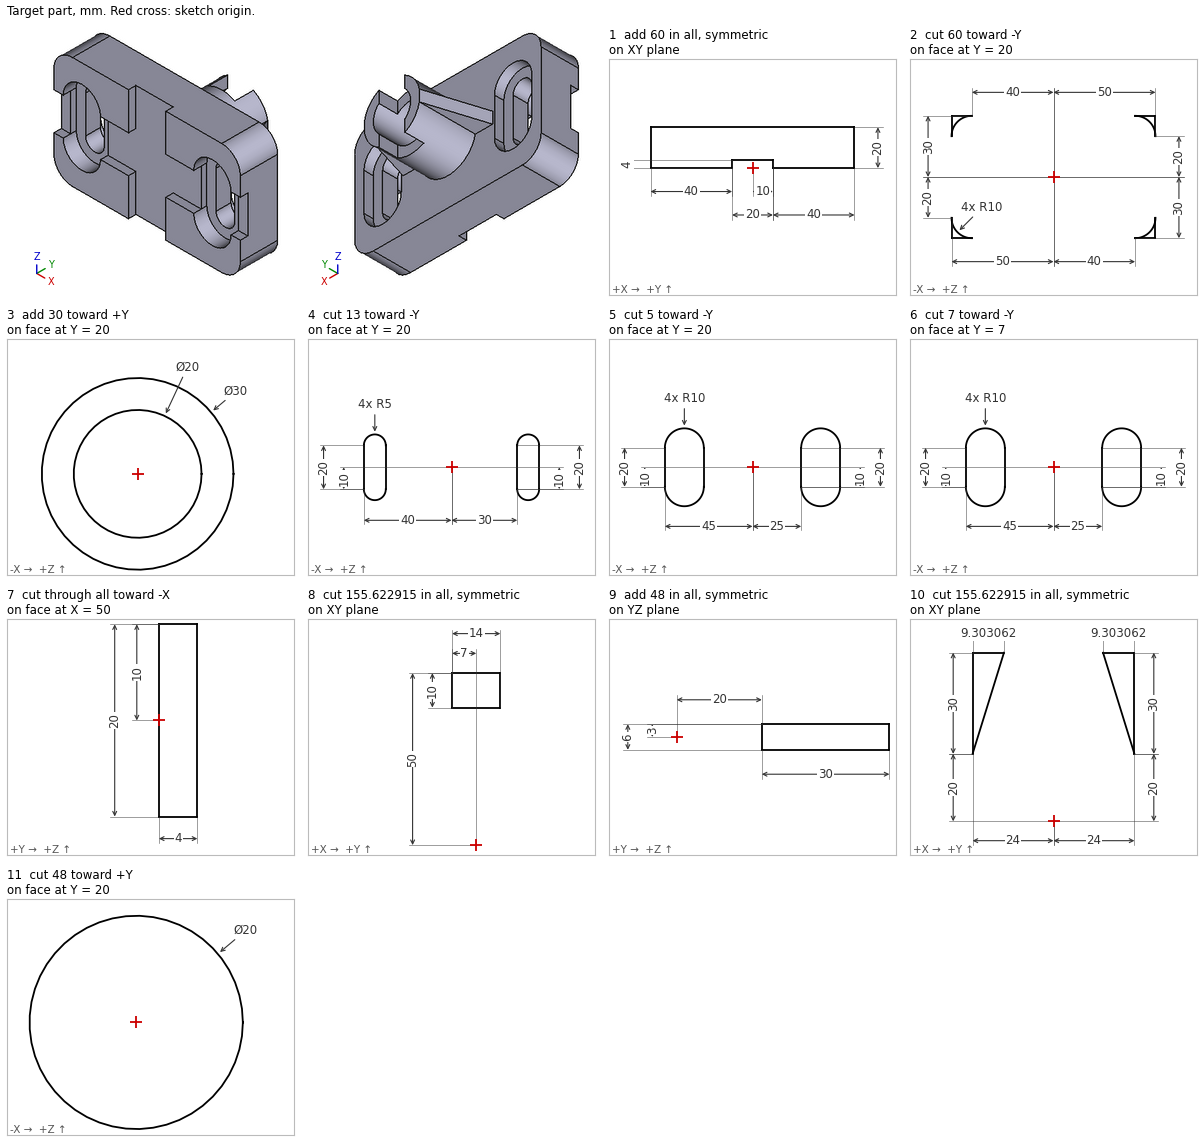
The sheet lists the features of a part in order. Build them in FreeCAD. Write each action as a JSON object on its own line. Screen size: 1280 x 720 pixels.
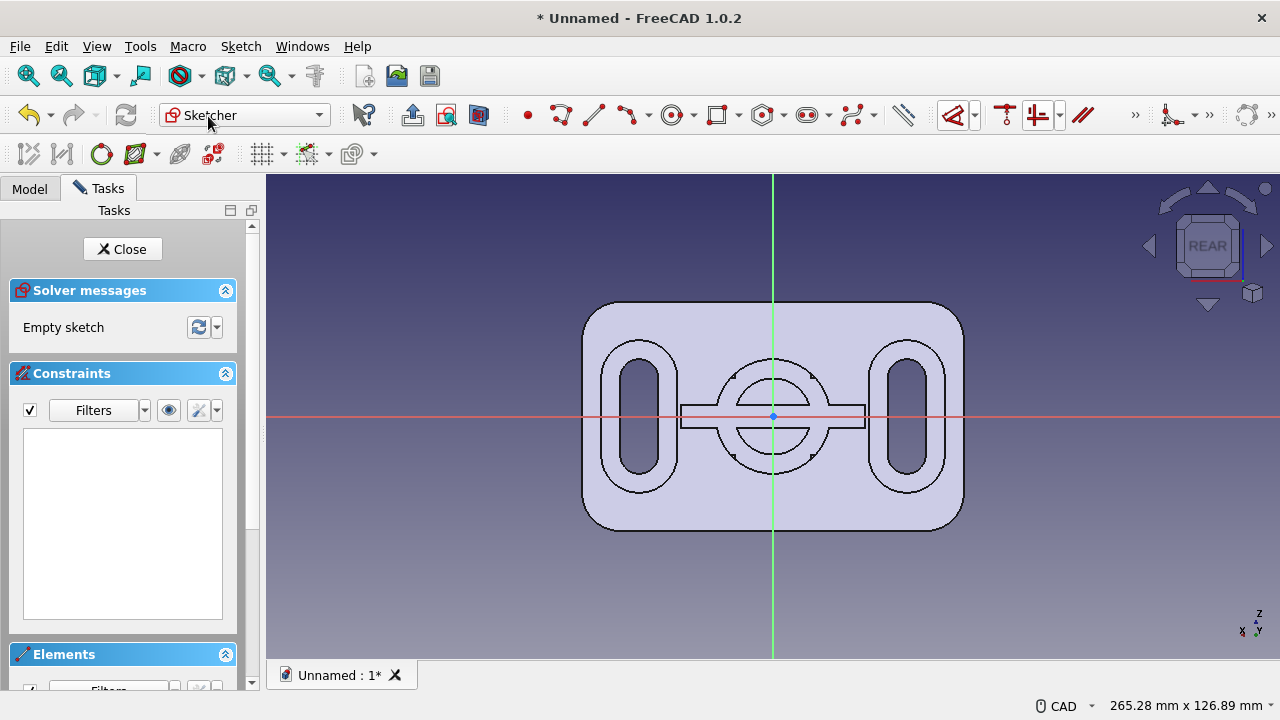
{"action": "scroll", "coordinate": [795, 416], "scroll_direction": "up", "scroll_amount": 7}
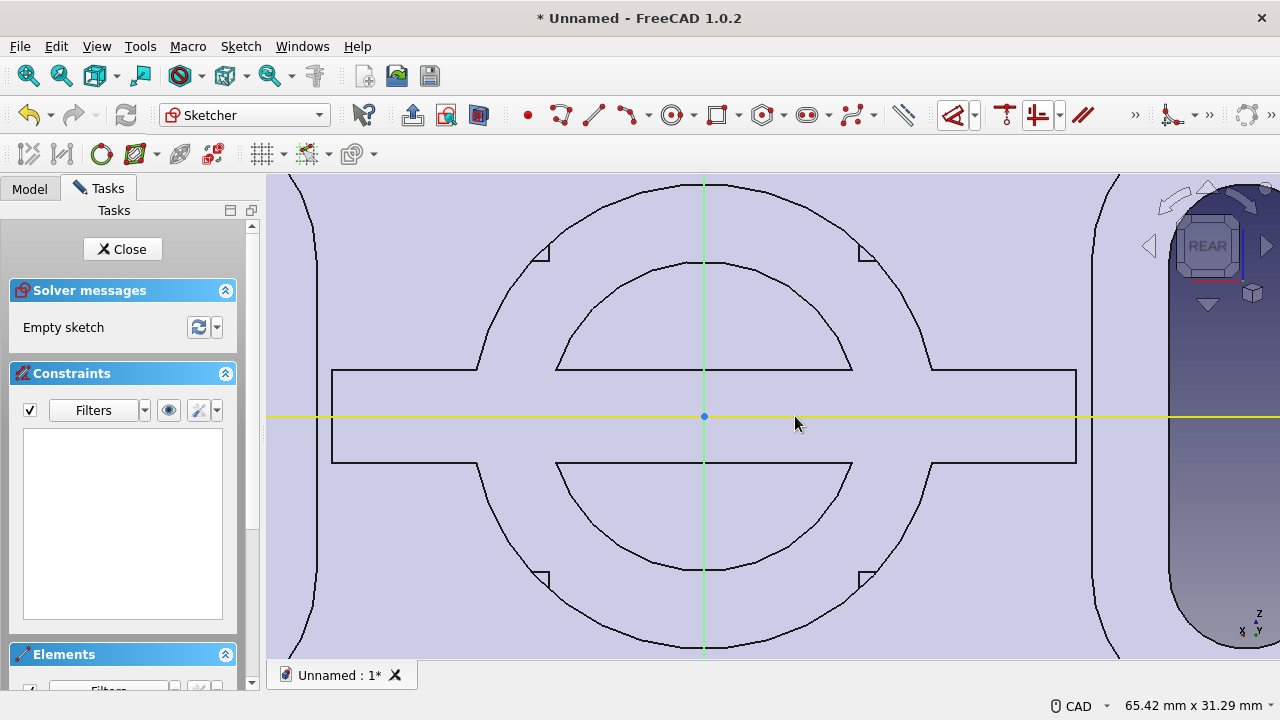
{"action": "key", "text": "g c"}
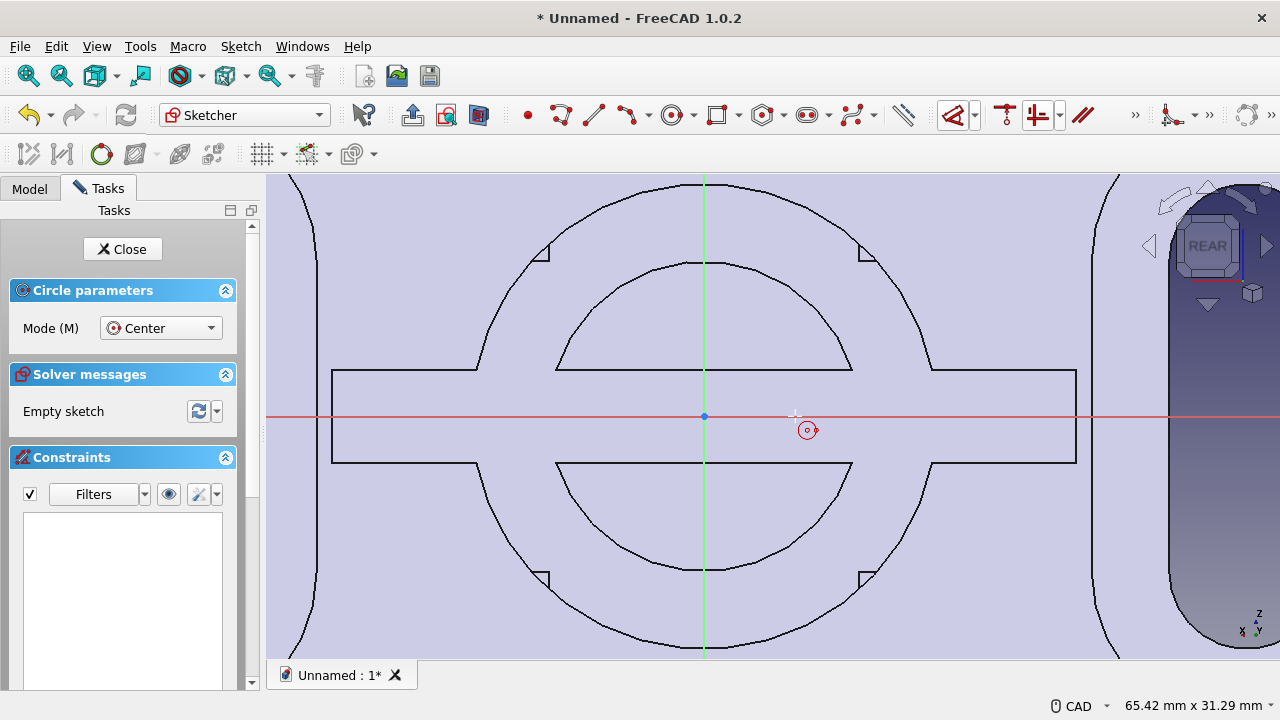
{"action": "left_click", "coordinate": [704, 416]}
{"action": "left_click", "coordinate": [814, 307]}
{"action": "key", "text": "Escape"}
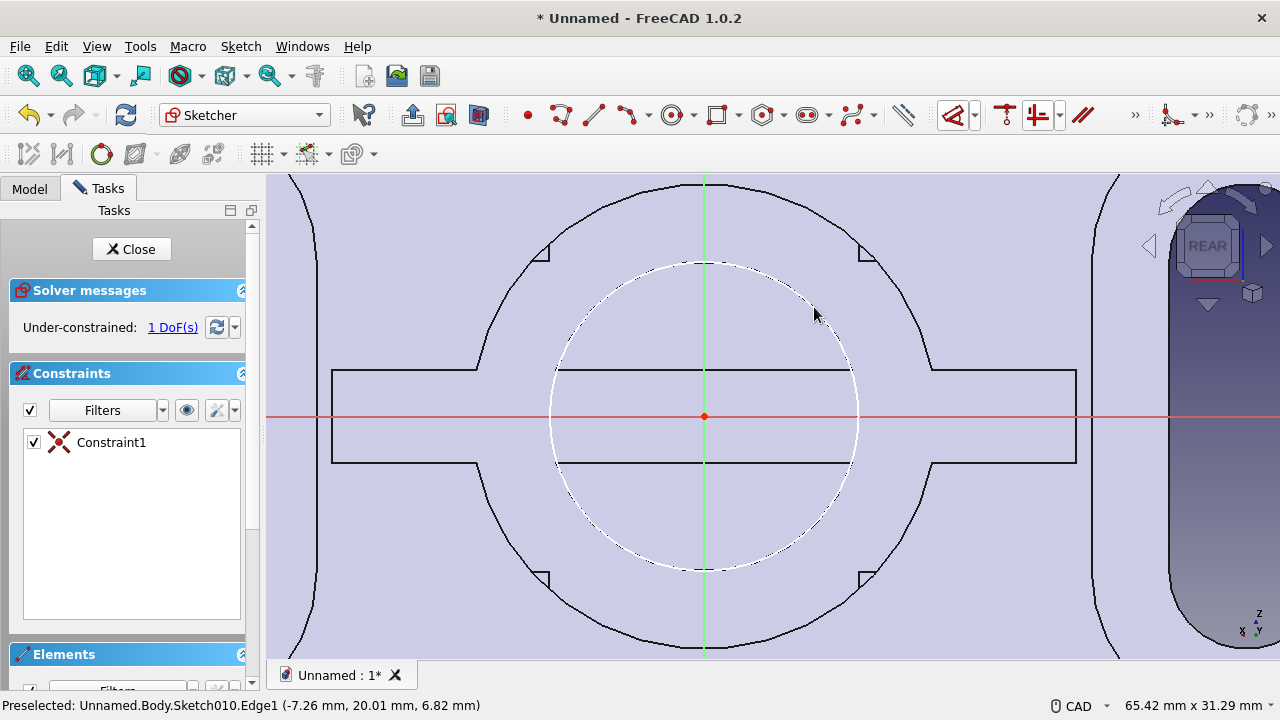
{"action": "left_click", "coordinate": [813, 307]}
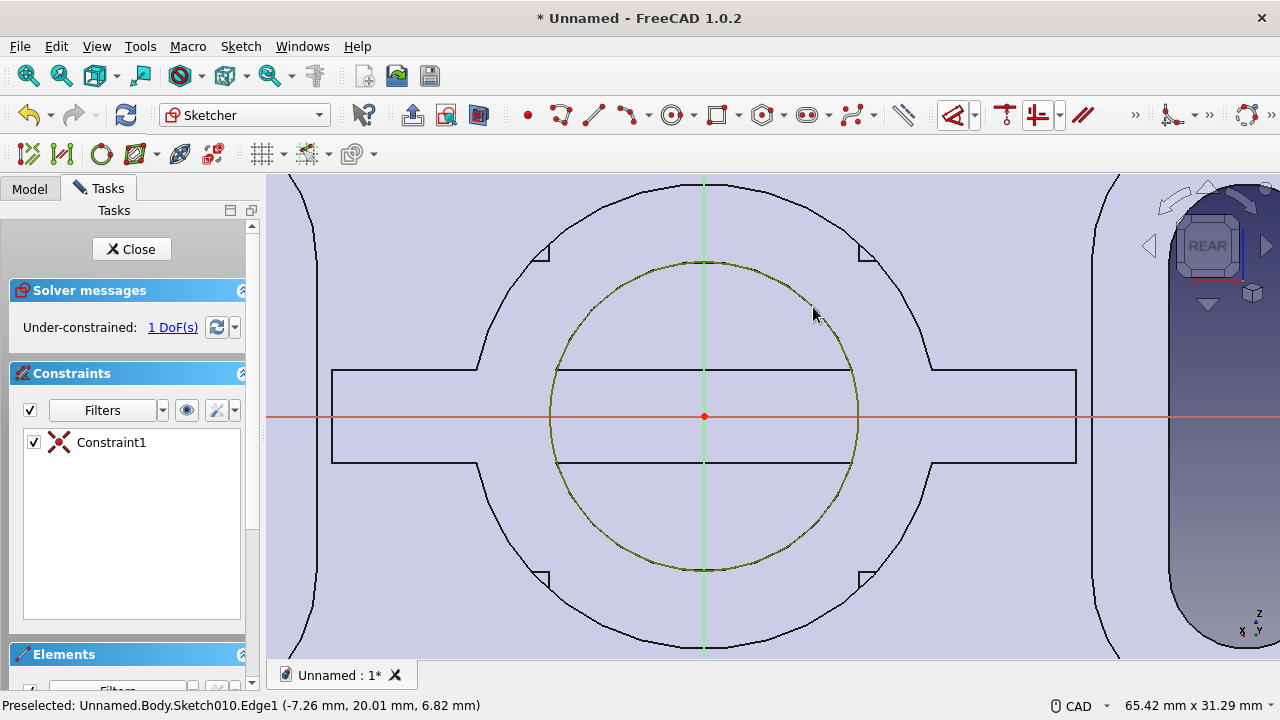
{"action": "left_click", "coordinate": [974, 116]}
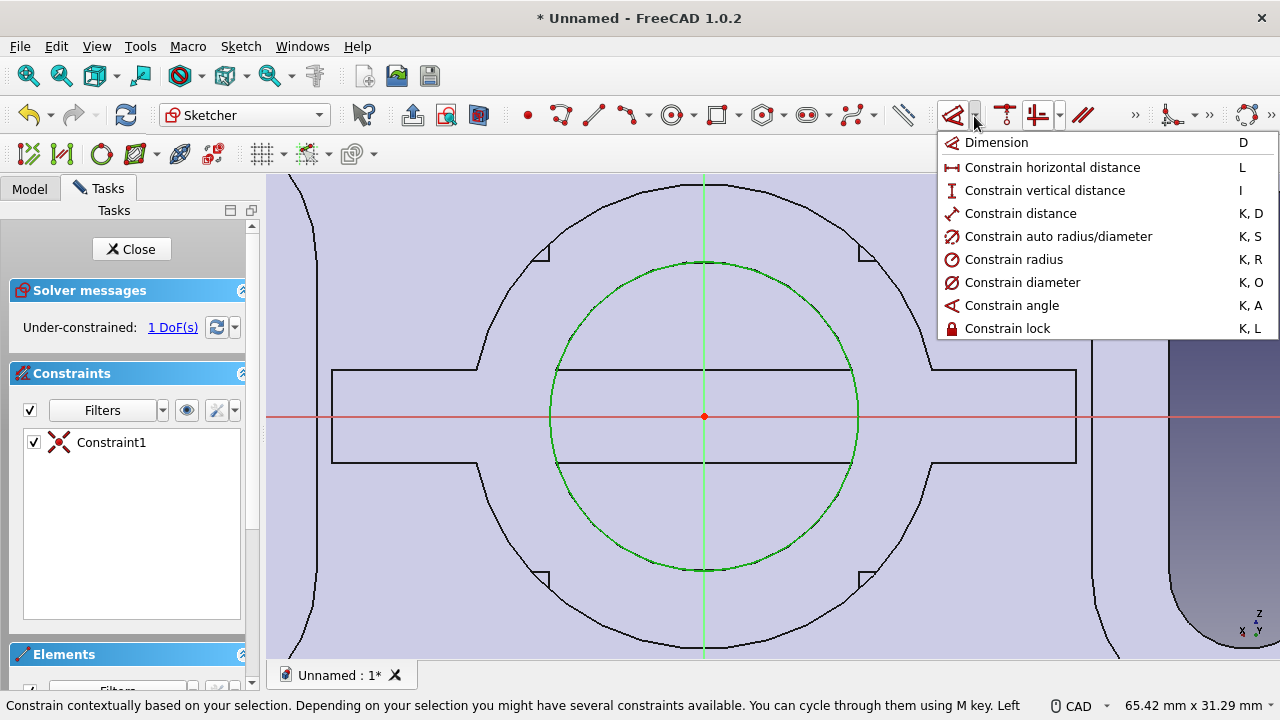
{"action": "left_click", "coordinate": [1108, 282]}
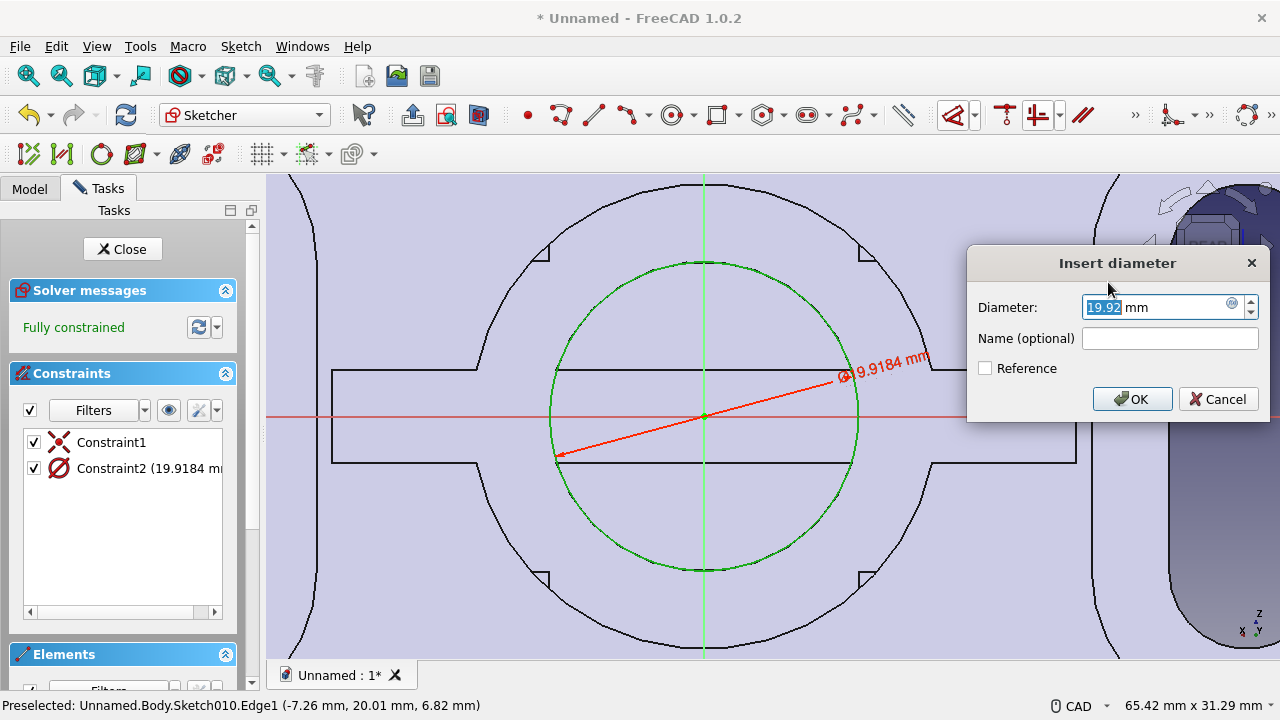
{"action": "type", "text": "20"}
{"action": "key", "text": "Return"}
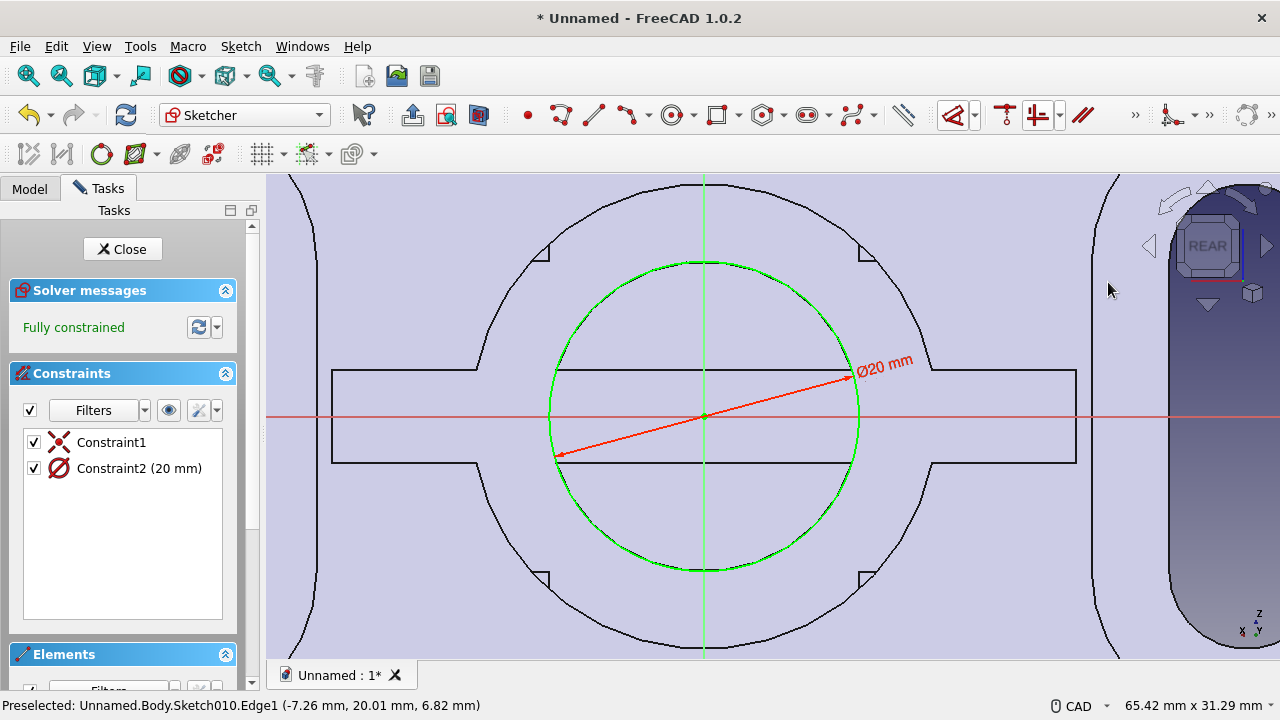
{"action": "left_click", "coordinate": [123, 249]}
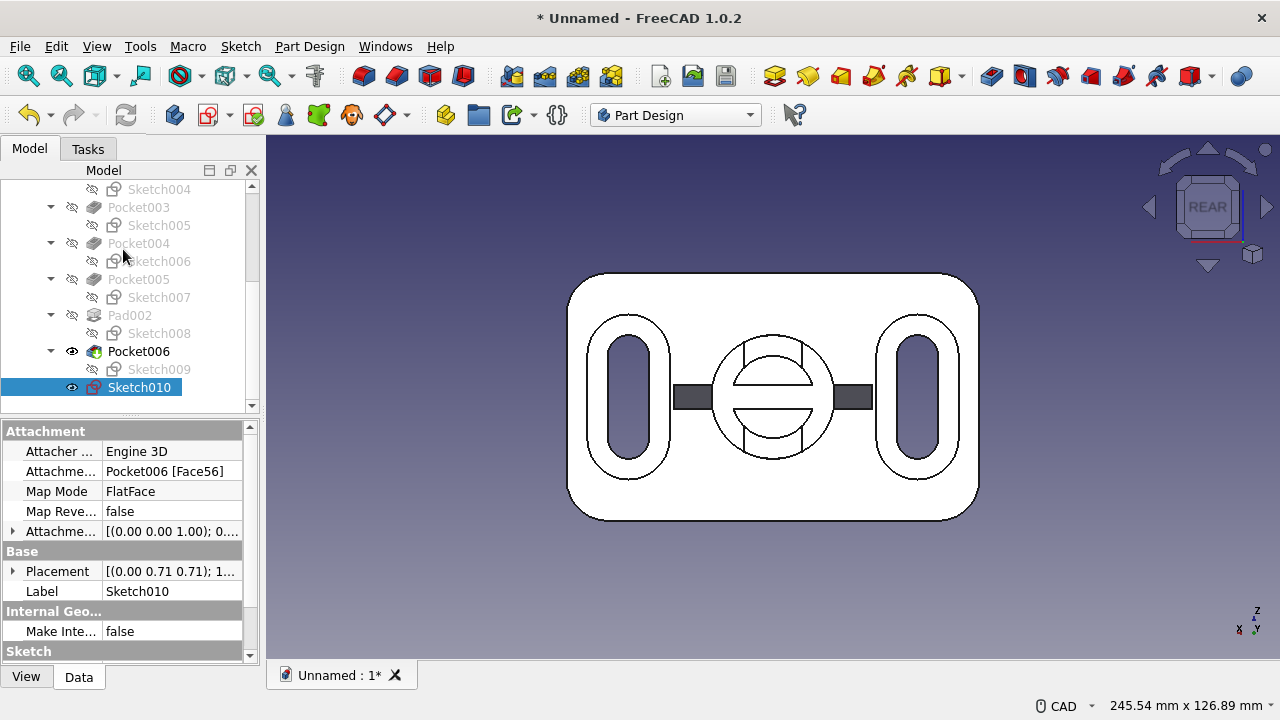
{"action": "left_click", "coordinate": [992, 76]}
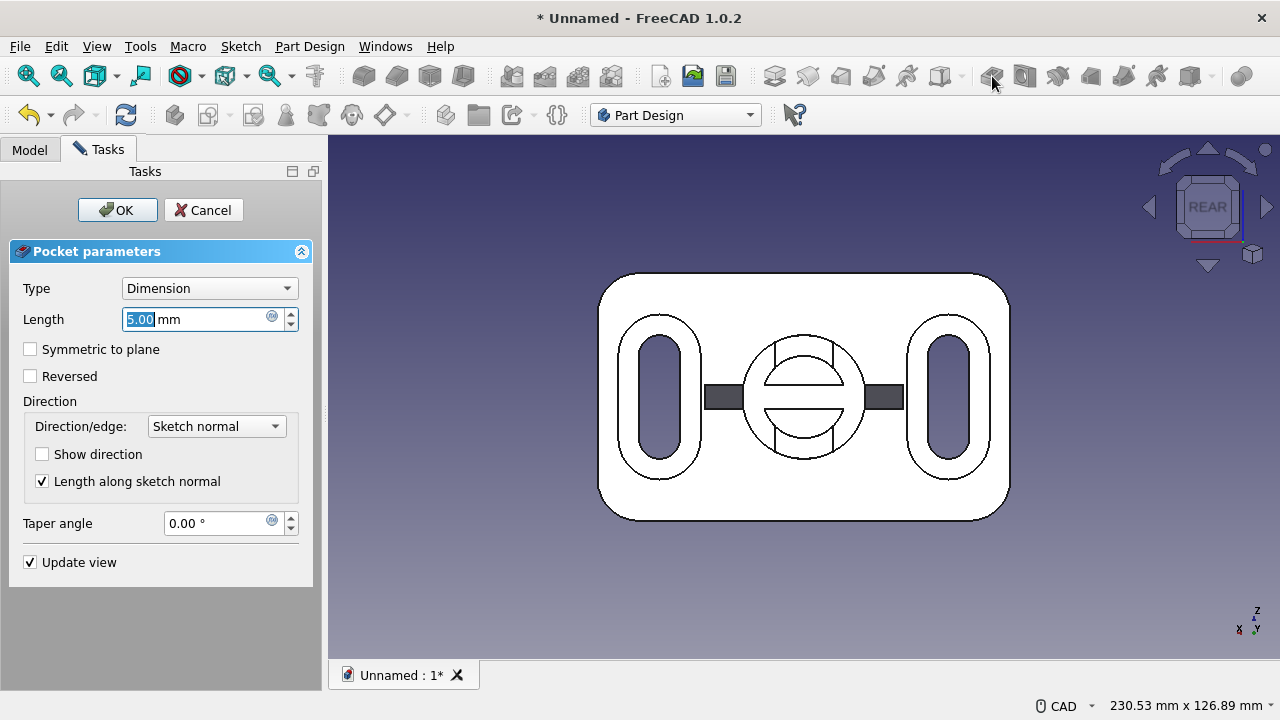
{"action": "type", "text": "48"}
{"action": "key", "text": "Tab"}